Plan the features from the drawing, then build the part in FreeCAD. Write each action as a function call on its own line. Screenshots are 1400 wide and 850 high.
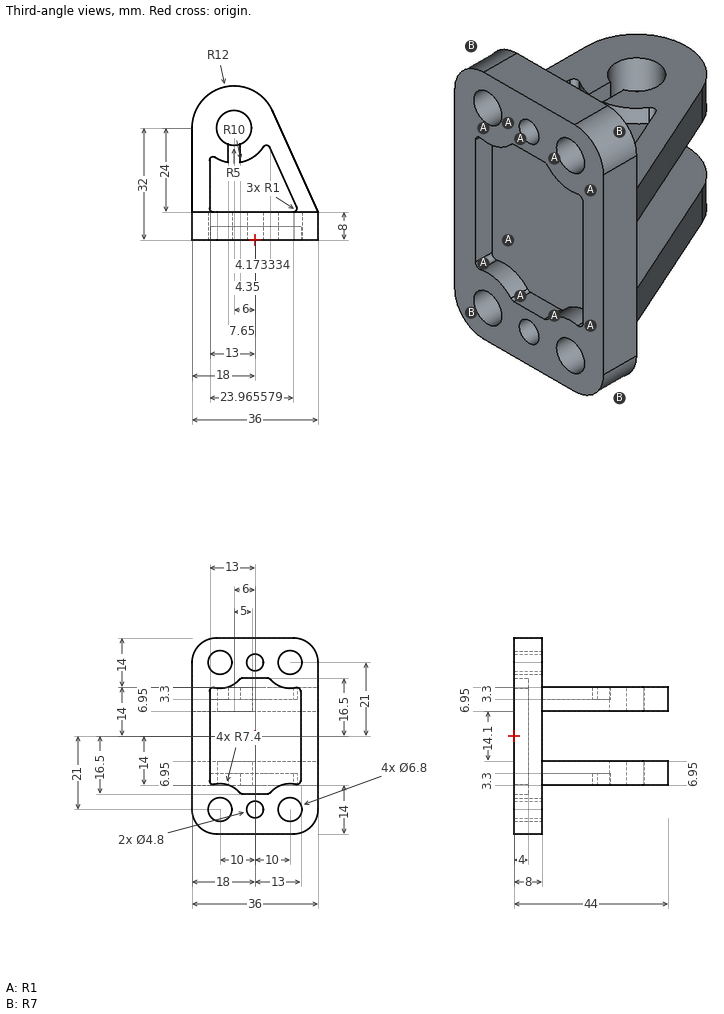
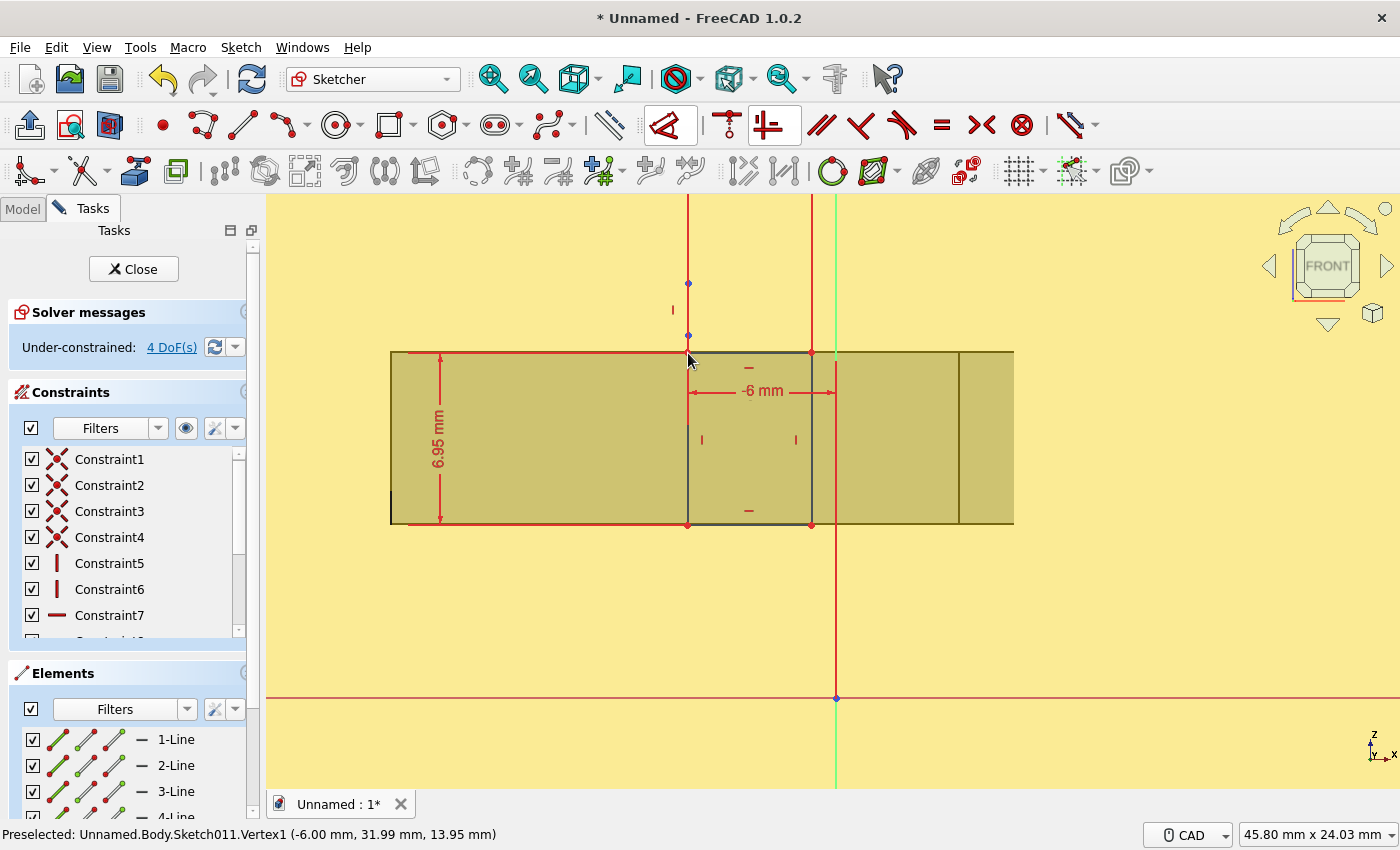
click(688, 336)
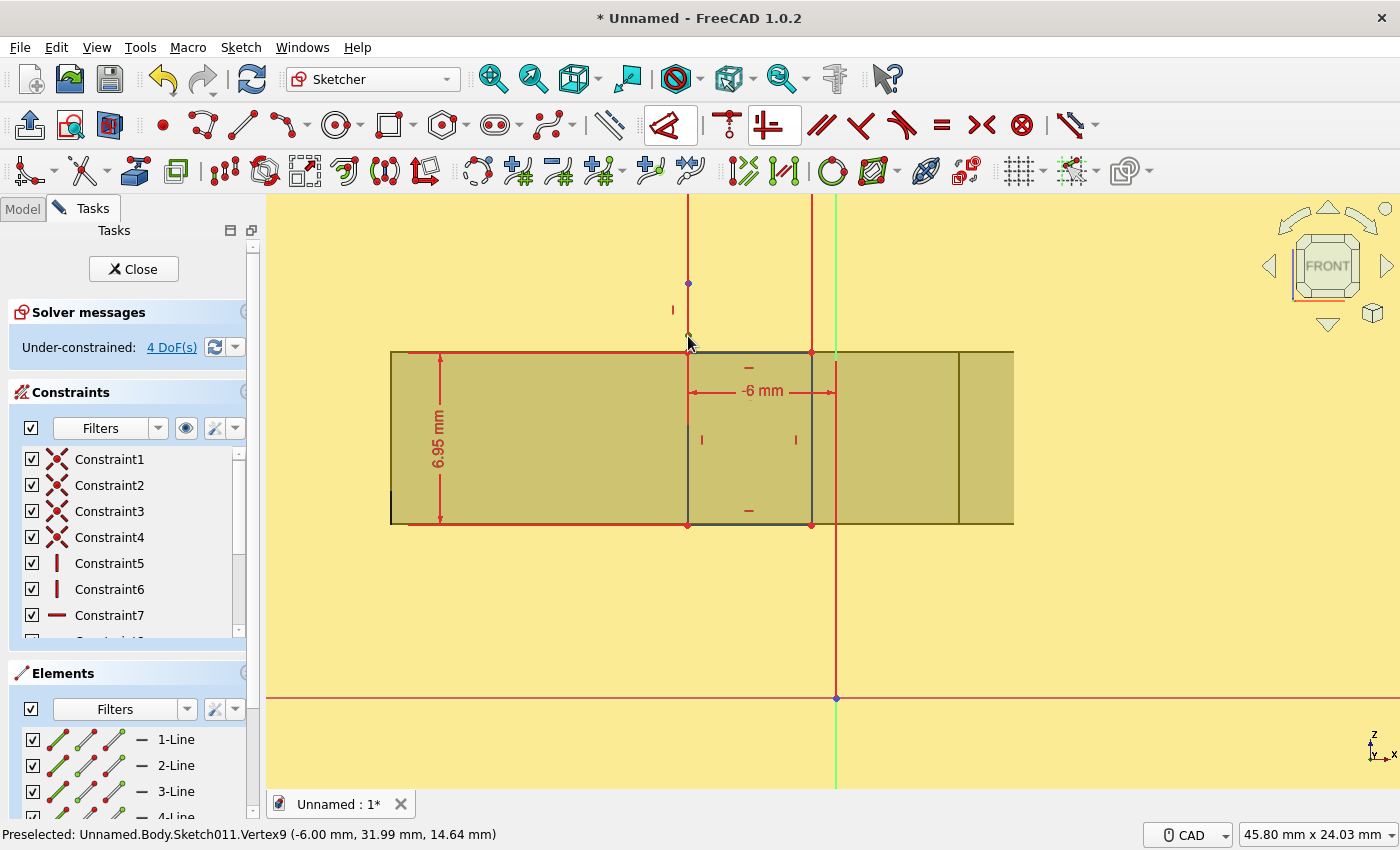
key(l)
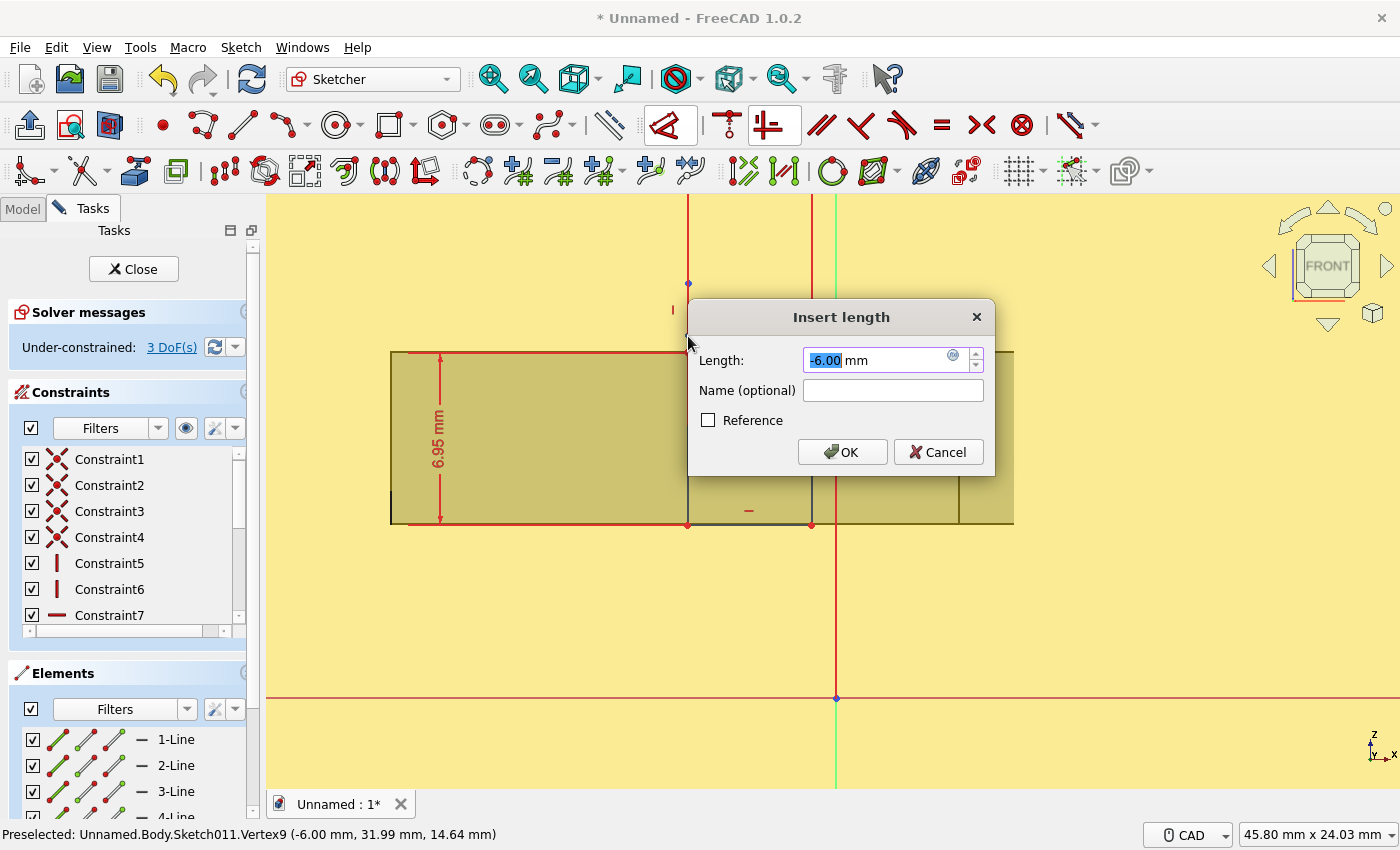
text(-6)
key(Return)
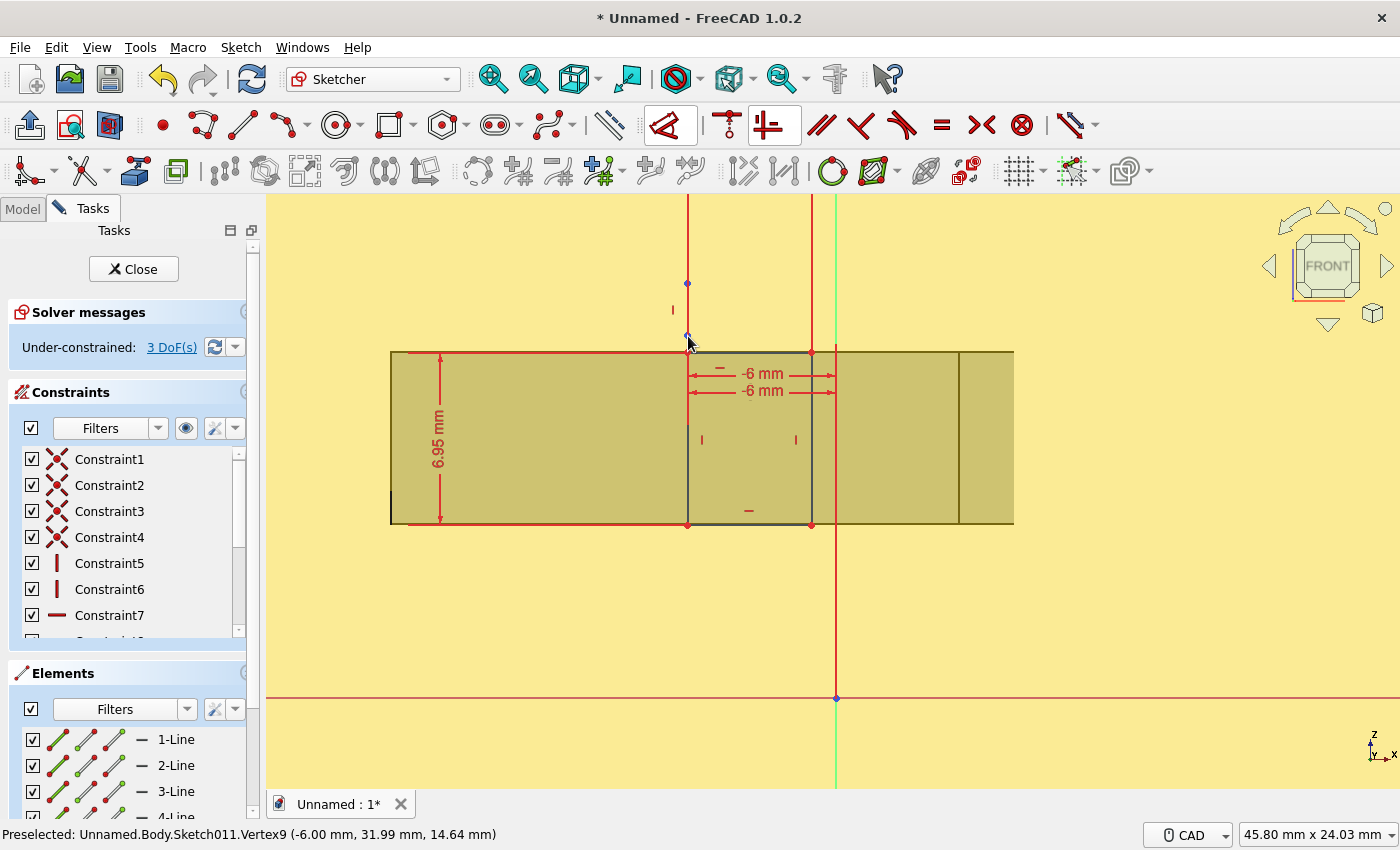
click(688, 353)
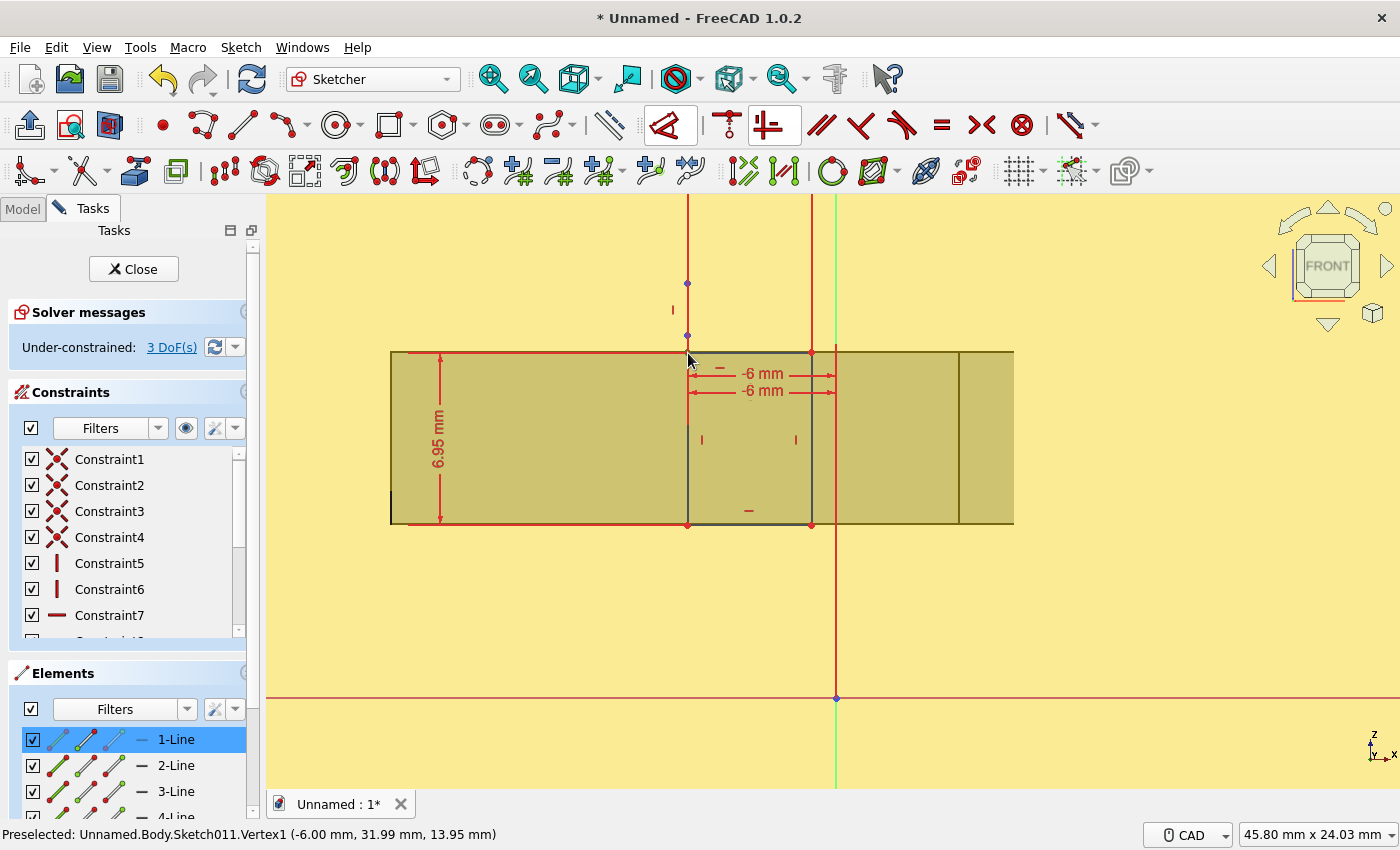
key(i)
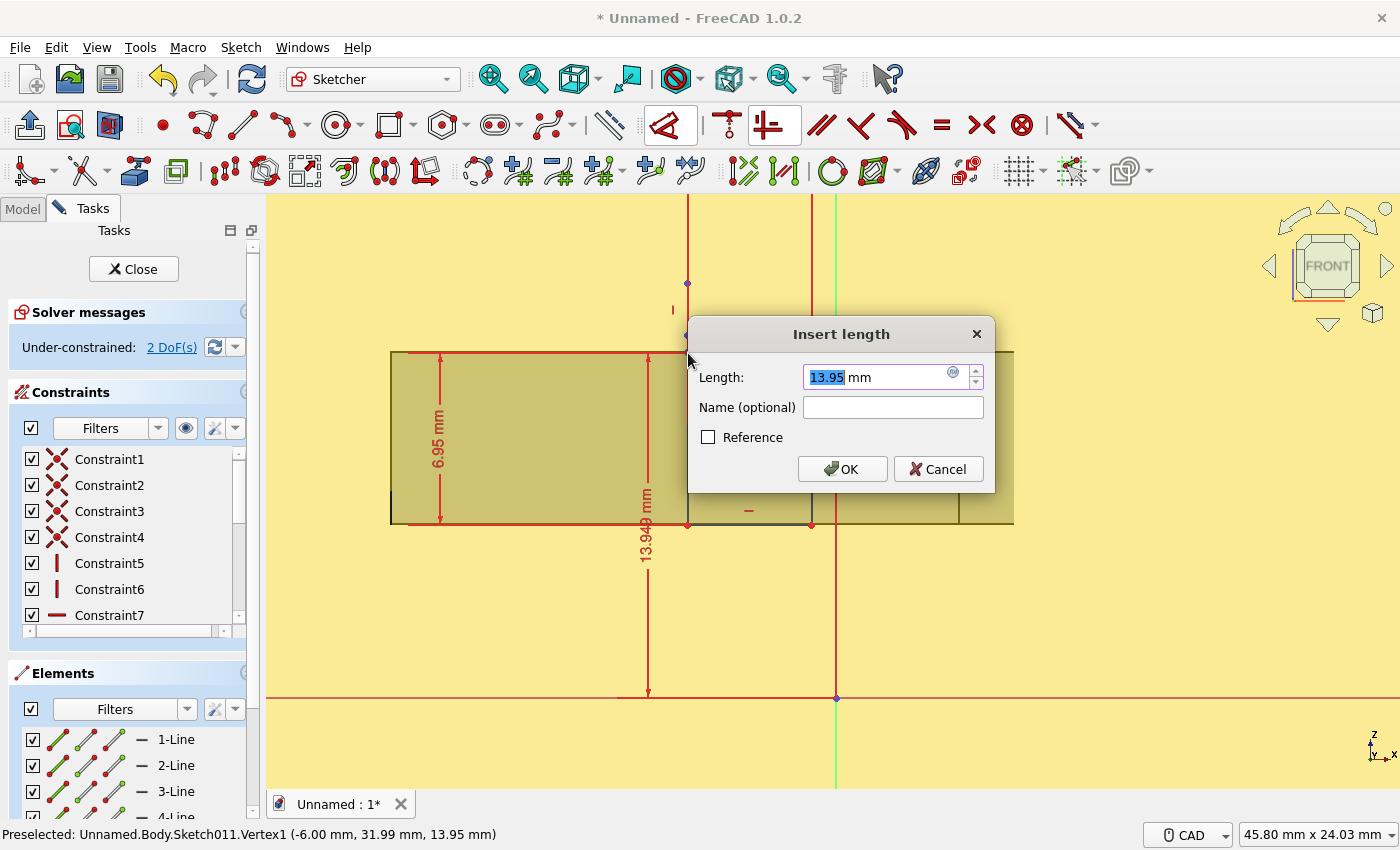
text(14)
key(Return)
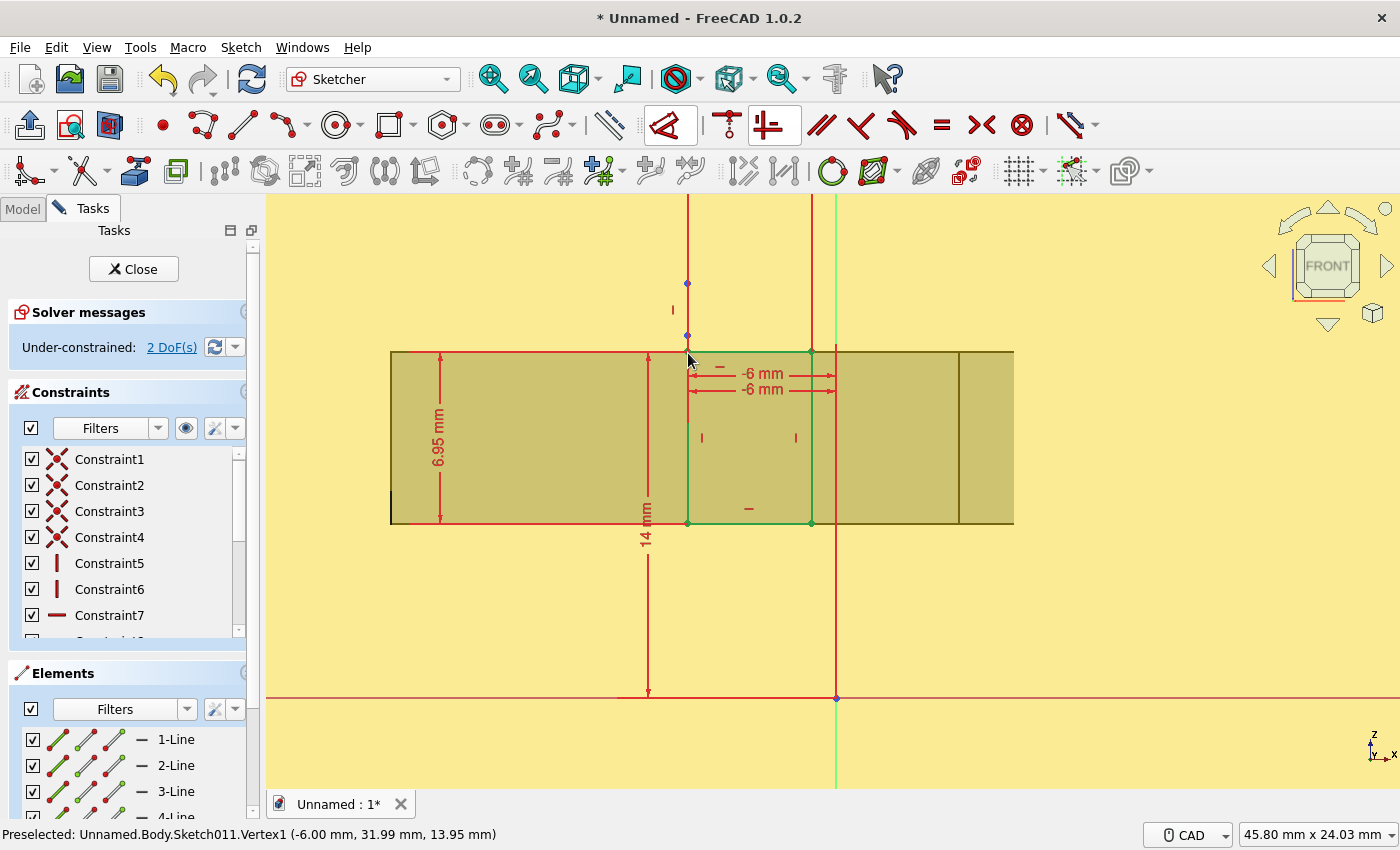
click(134, 269)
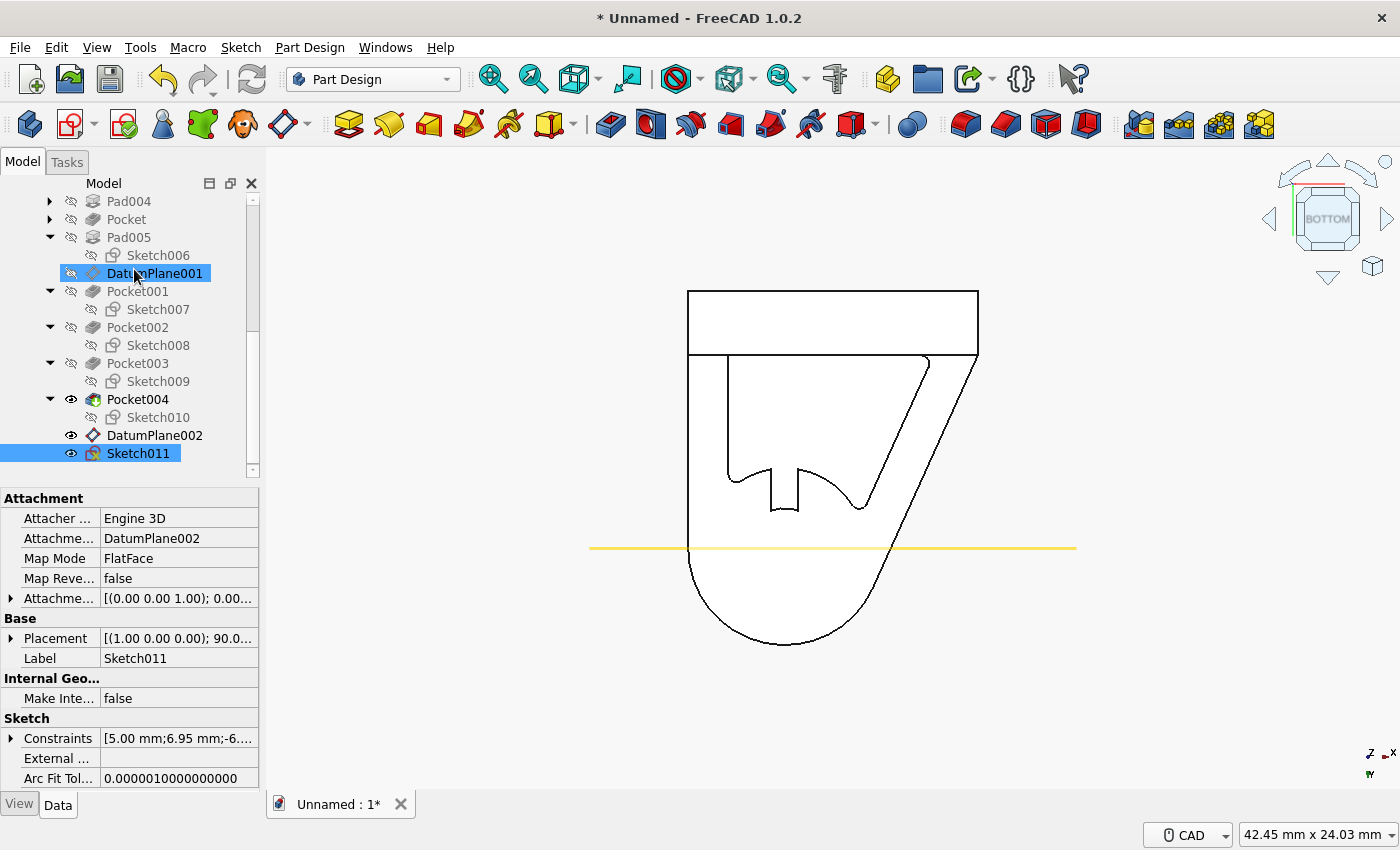
click(692, 124)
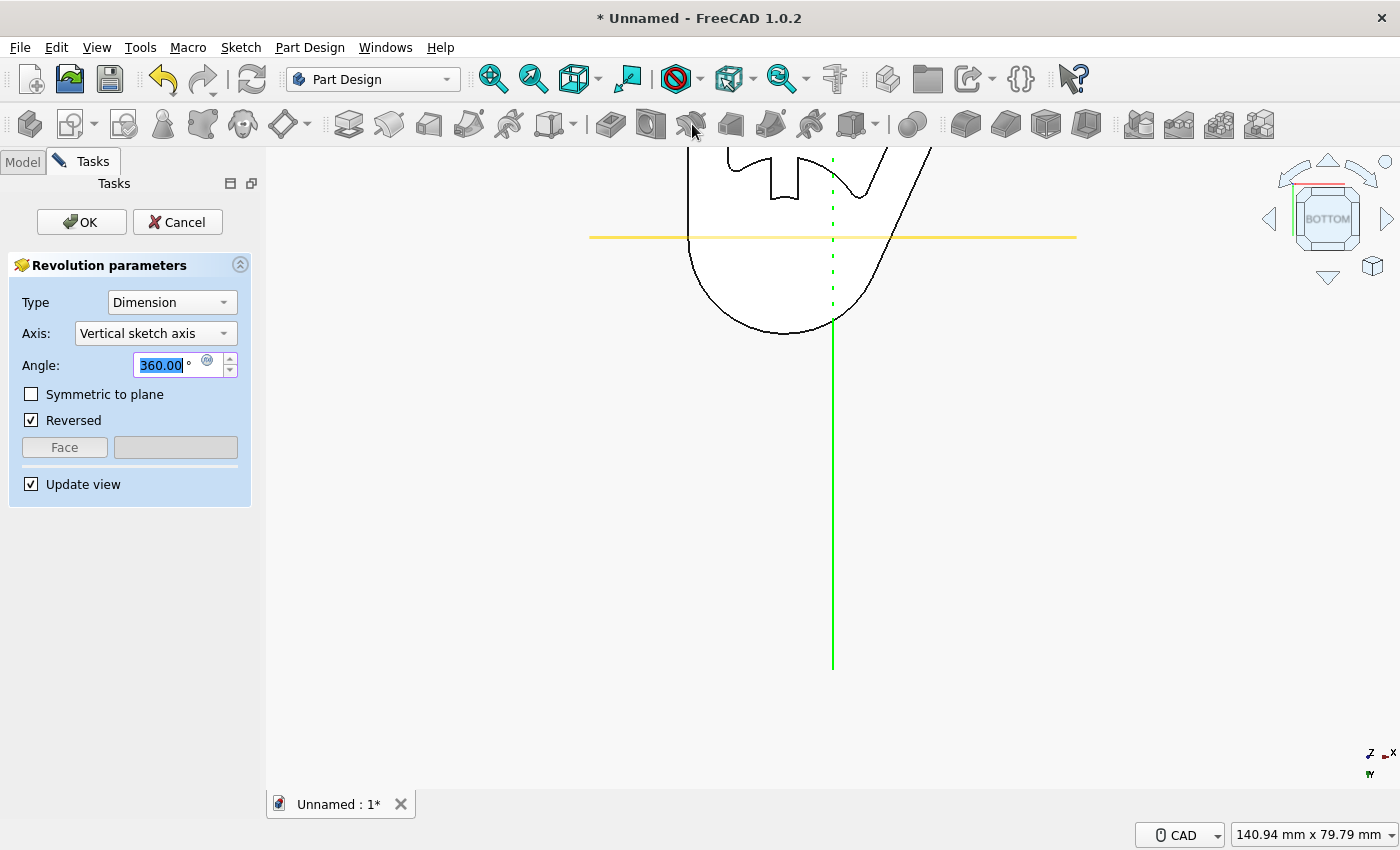
click(156, 334)